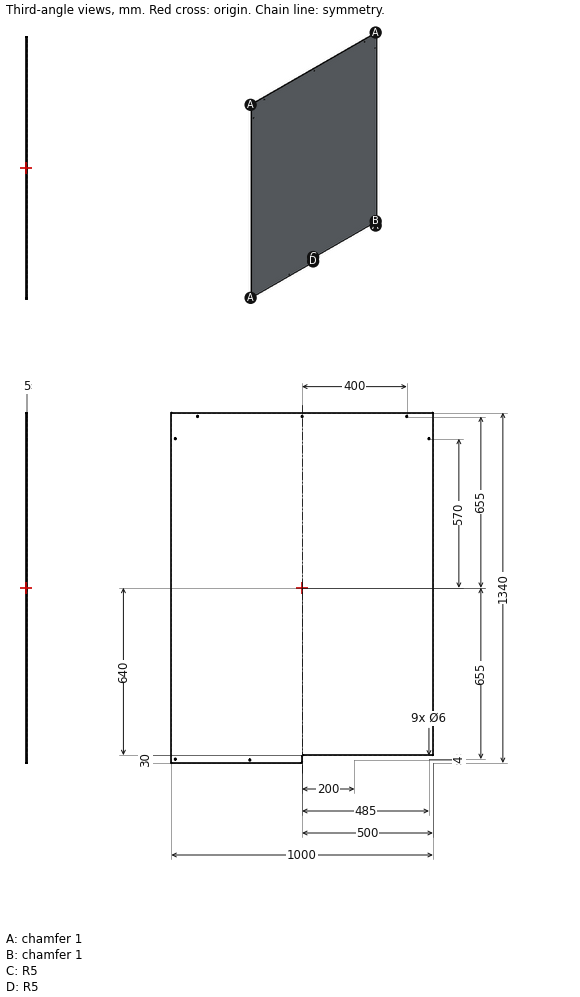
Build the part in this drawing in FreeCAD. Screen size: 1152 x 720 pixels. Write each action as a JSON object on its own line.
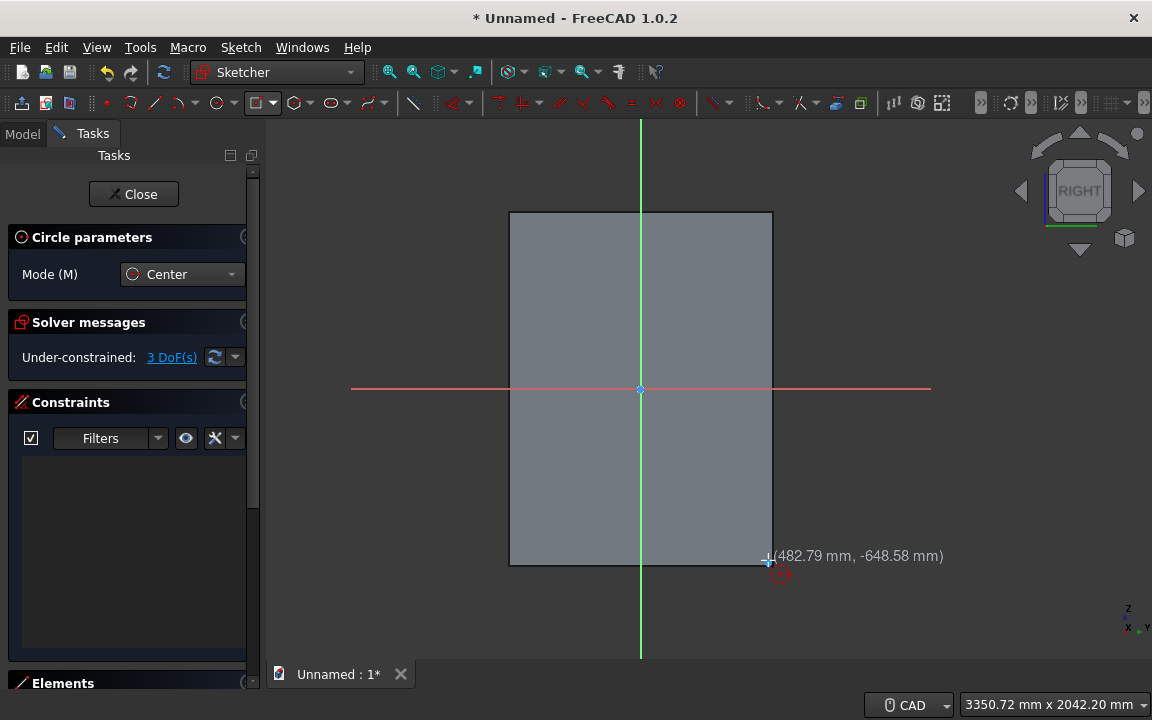
{"action": "scroll", "coordinate": [513, 563], "scroll_direction": "up", "scroll_amount": 17}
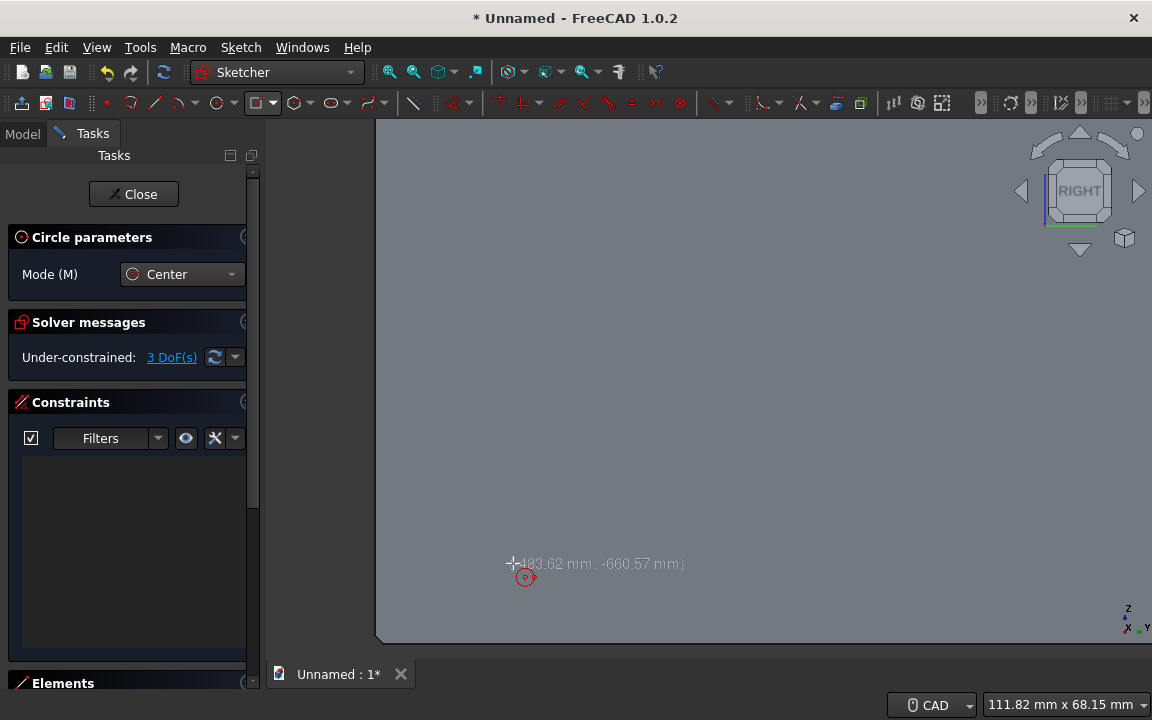
{"action": "scroll", "coordinate": [483, 603], "scroll_direction": "down", "scroll_amount": 16}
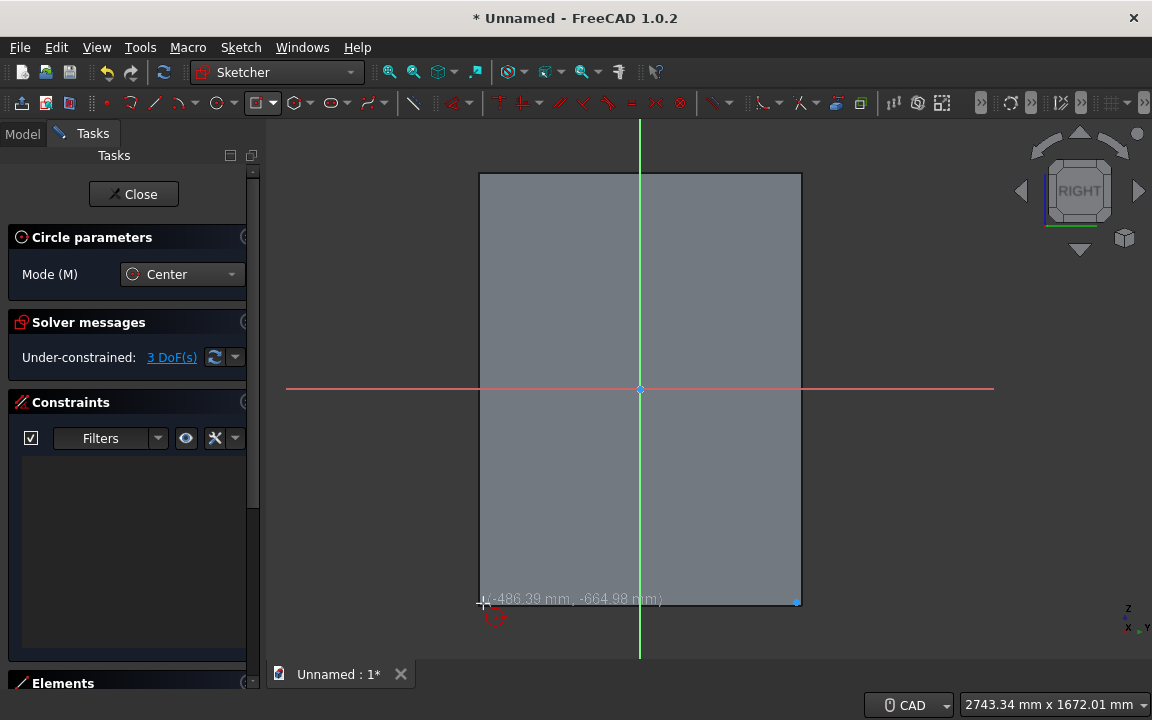
{"action": "left_click", "coordinate": [484, 601]}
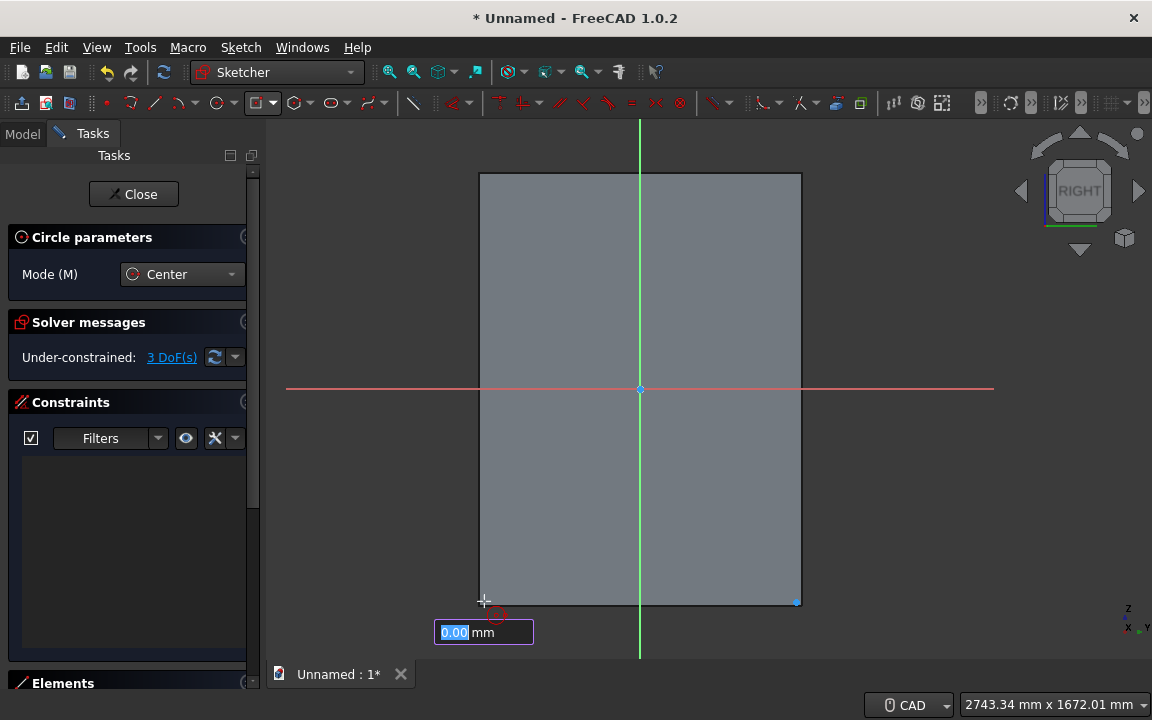
{"action": "scroll", "coordinate": [484, 600], "scroll_direction": "up", "scroll_amount": 14}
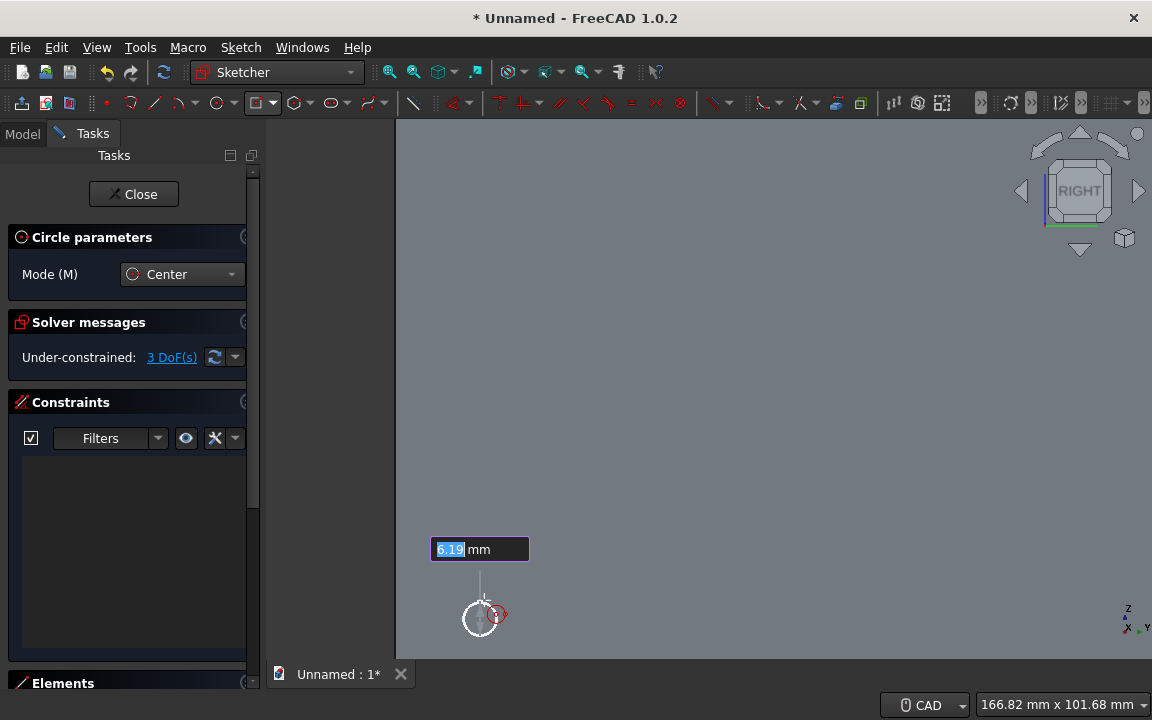
{"action": "left_click", "coordinate": [486, 586]}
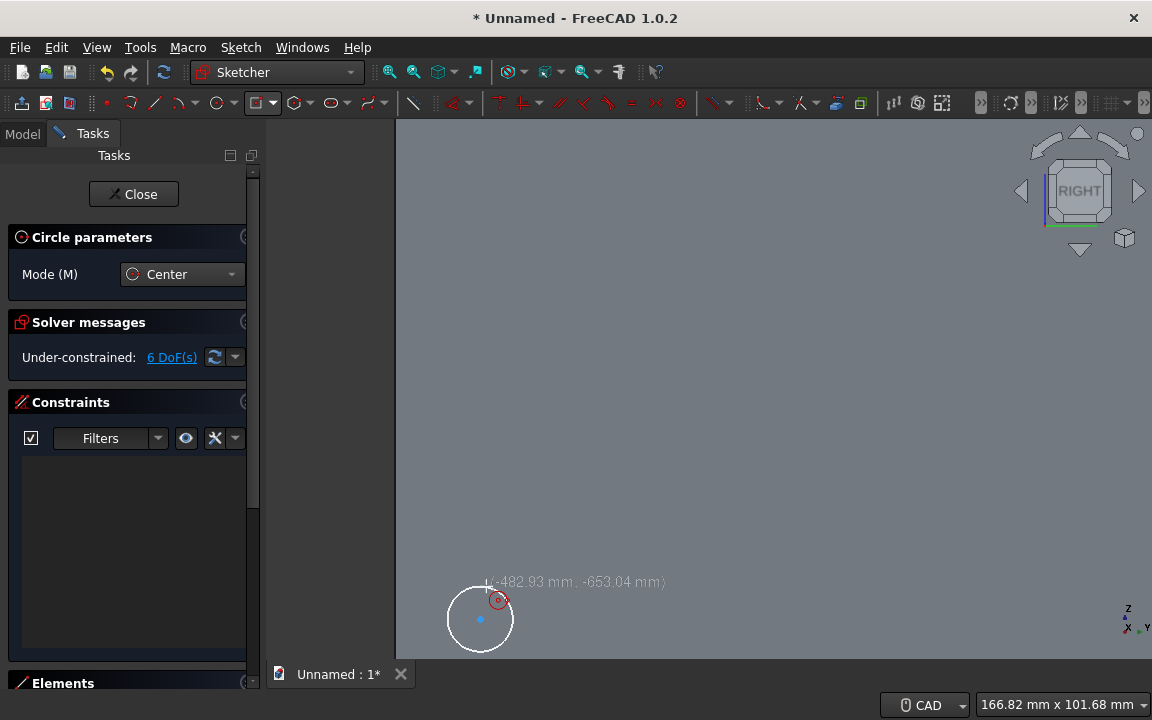
{"action": "scroll", "coordinate": [514, 560], "scroll_direction": "down", "scroll_amount": 15}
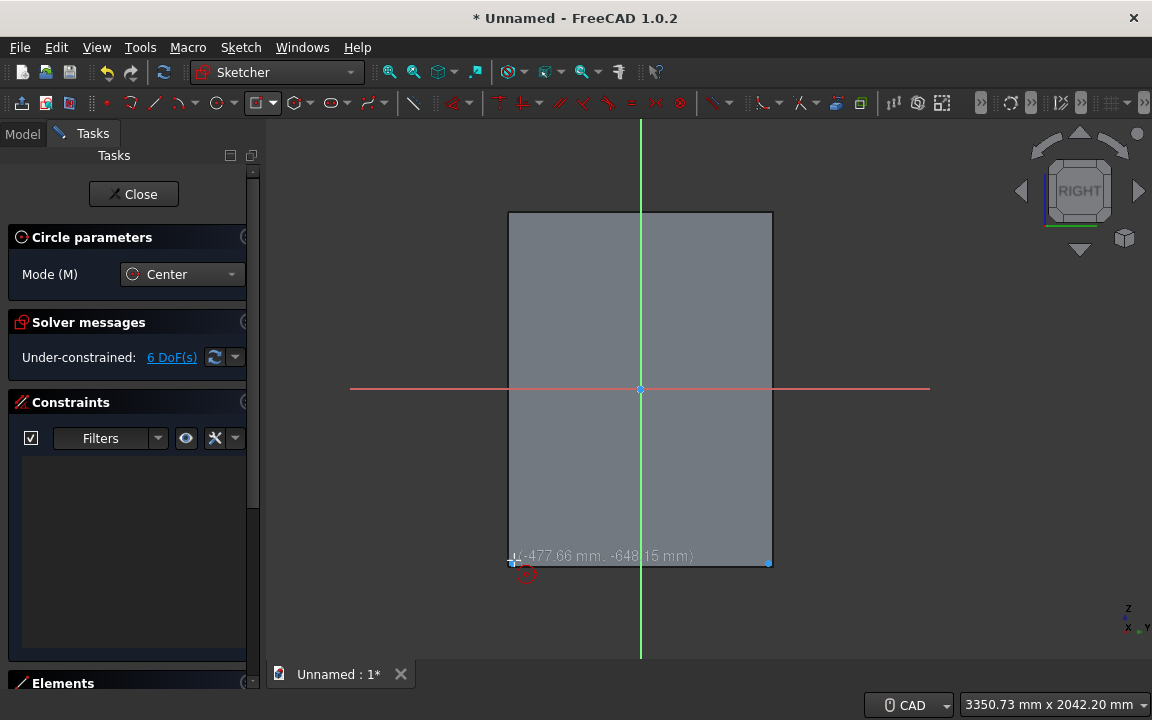
{"action": "scroll", "coordinate": [769, 239], "scroll_direction": "up", "scroll_amount": 17}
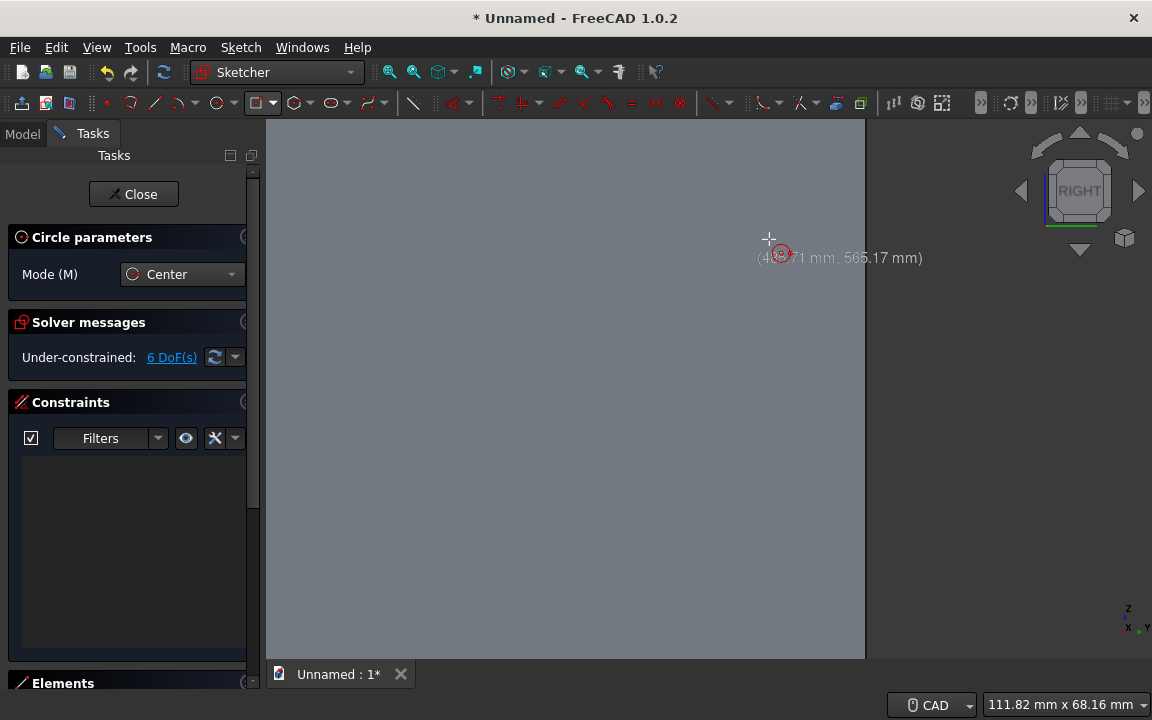
{"action": "scroll", "coordinate": [799, 203], "scroll_direction": "down", "scroll_amount": 16}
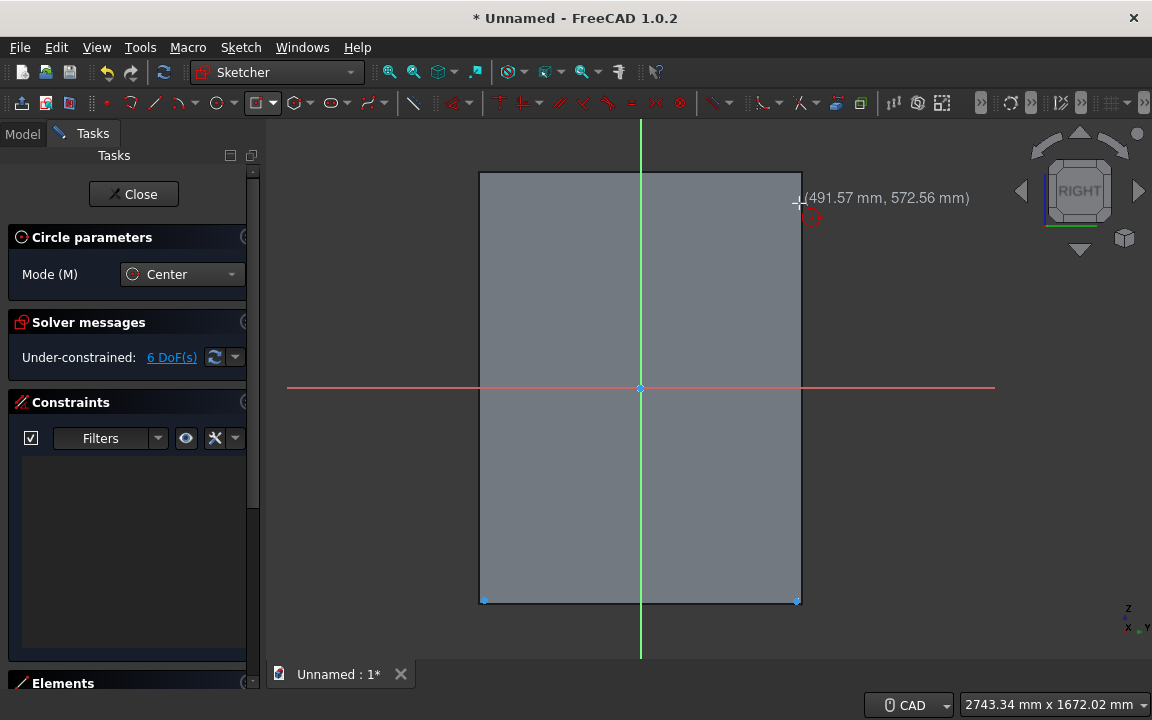
{"action": "left_click", "coordinate": [797, 204]}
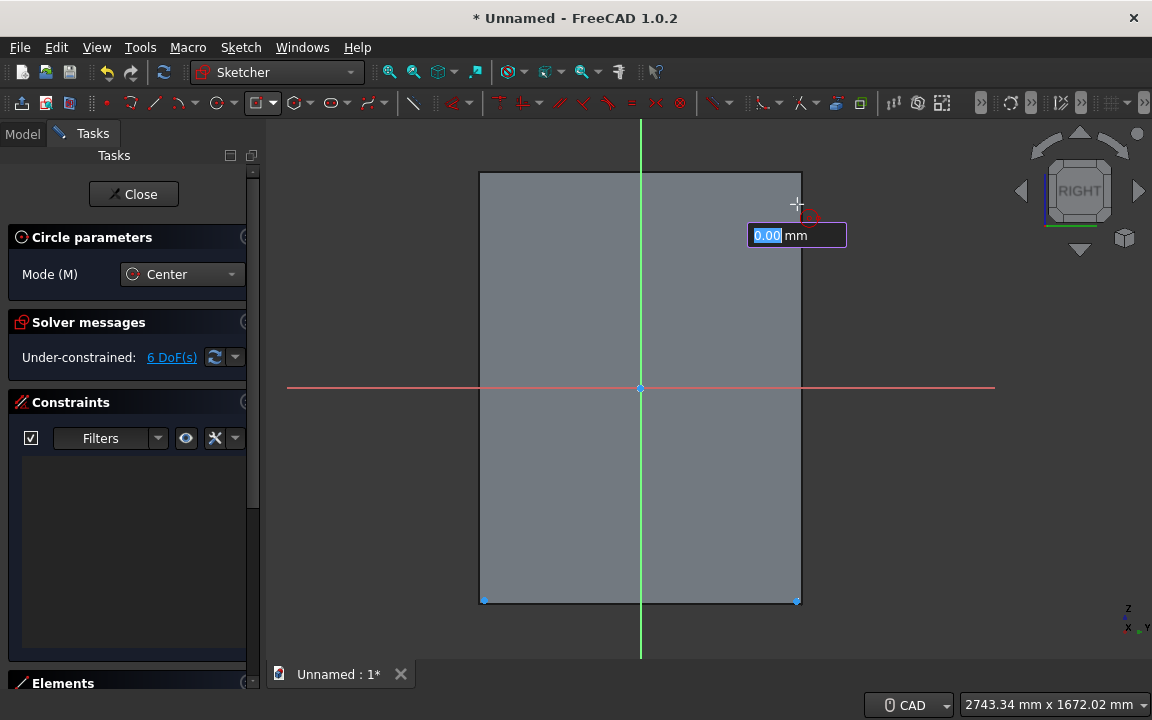
{"action": "scroll", "coordinate": [798, 203], "scroll_direction": "up", "scroll_amount": 14}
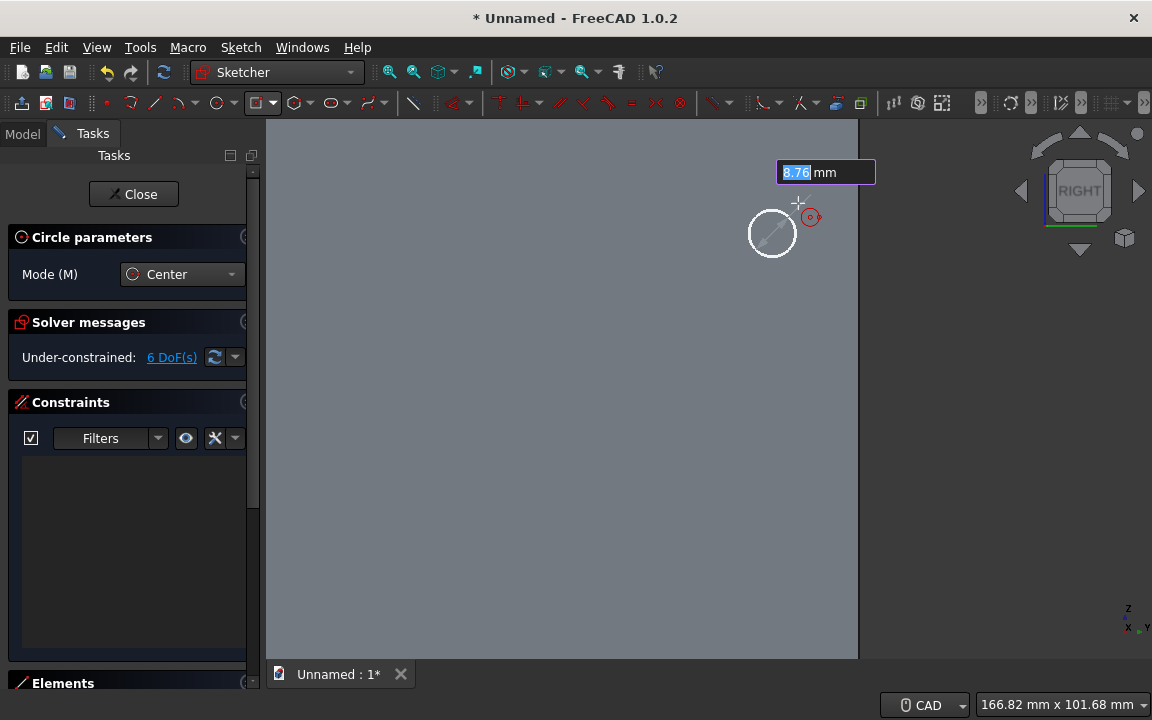
{"action": "left_click", "coordinate": [791, 206]}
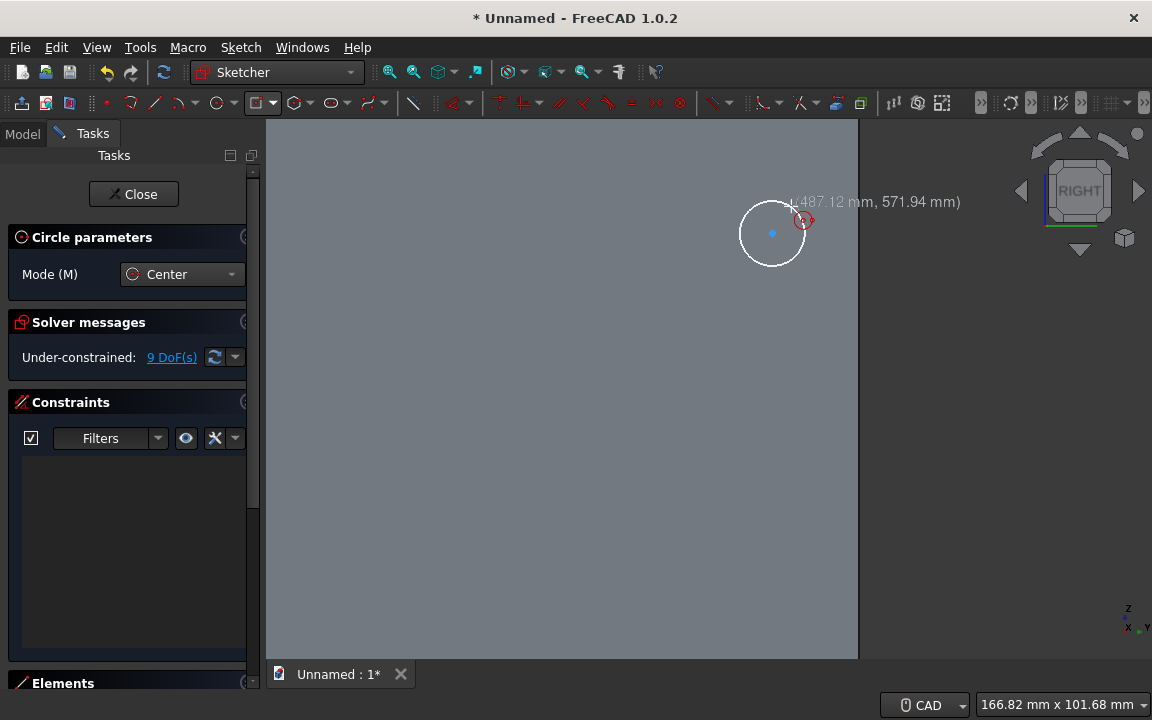
{"action": "scroll", "coordinate": [768, 239], "scroll_direction": "down", "scroll_amount": 15}